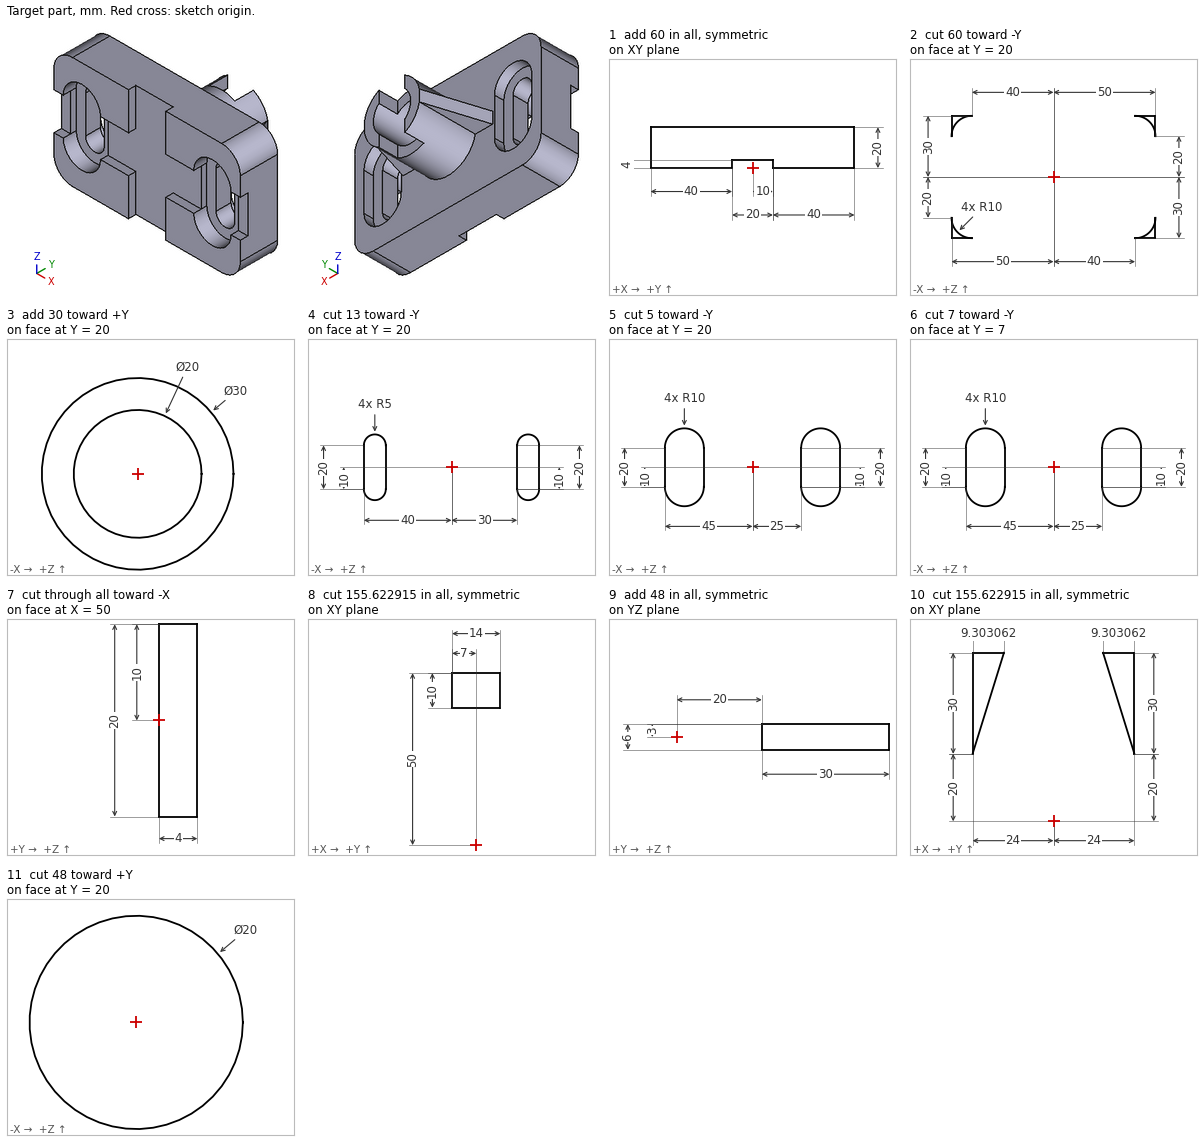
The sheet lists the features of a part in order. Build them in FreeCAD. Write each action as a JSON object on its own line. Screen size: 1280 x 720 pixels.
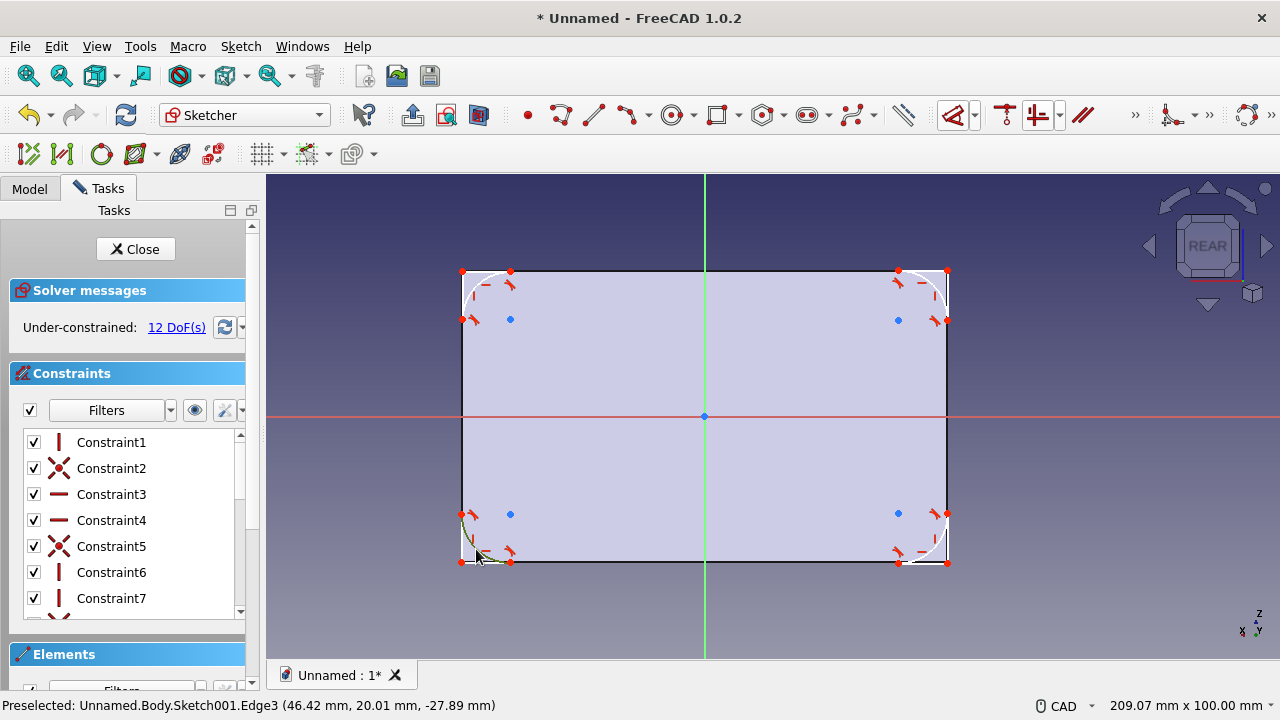
{"action": "left_click", "coordinate": [933, 549]}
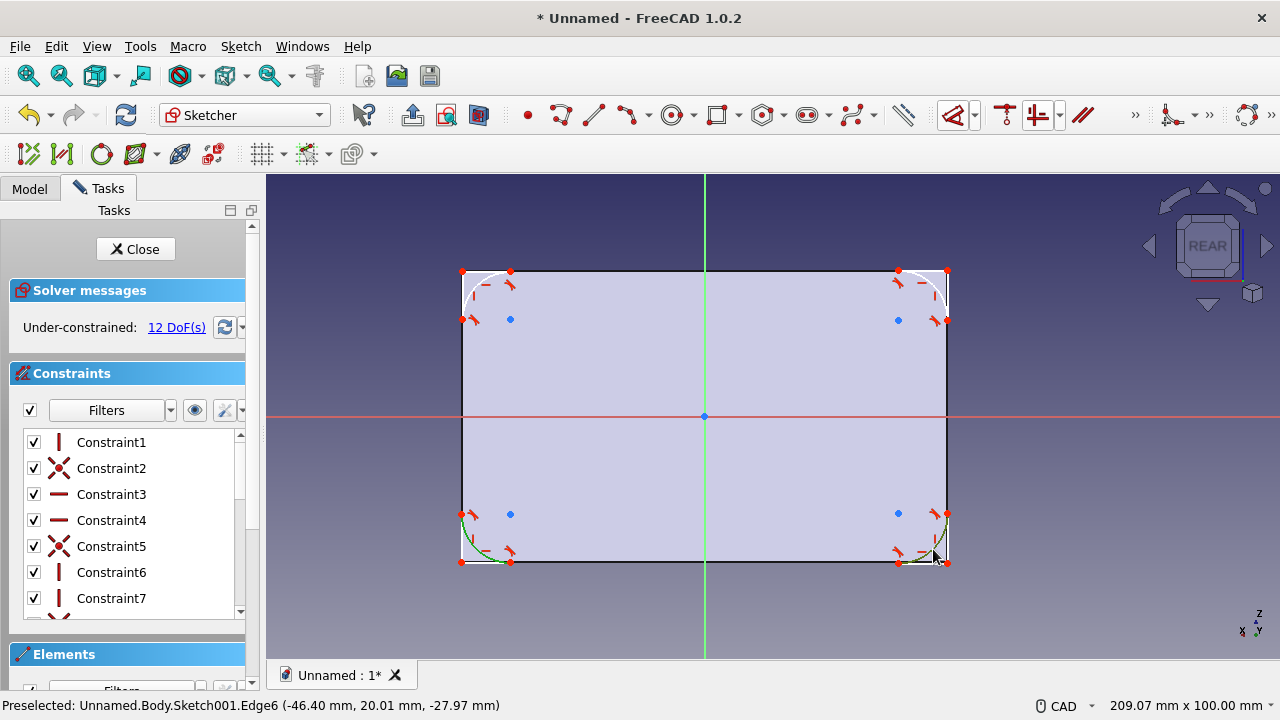
{"action": "left_click", "coordinate": [933, 285]}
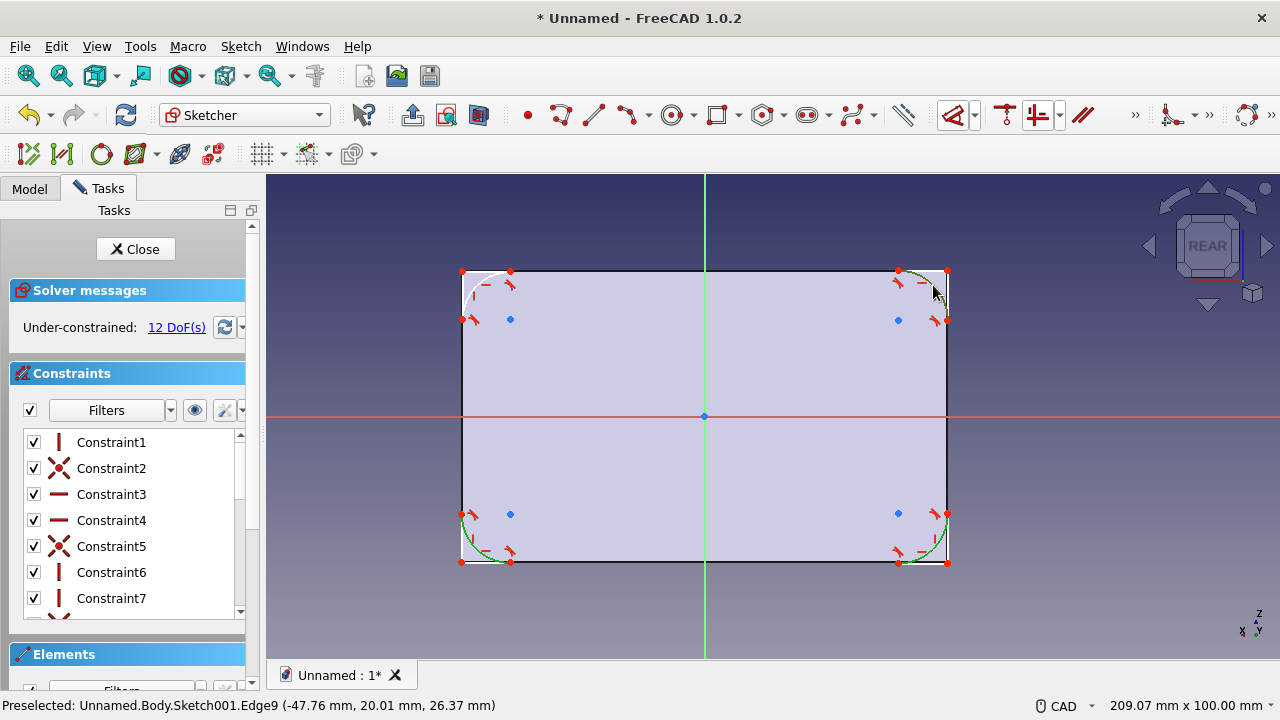
{"action": "left_click", "coordinate": [477, 286]}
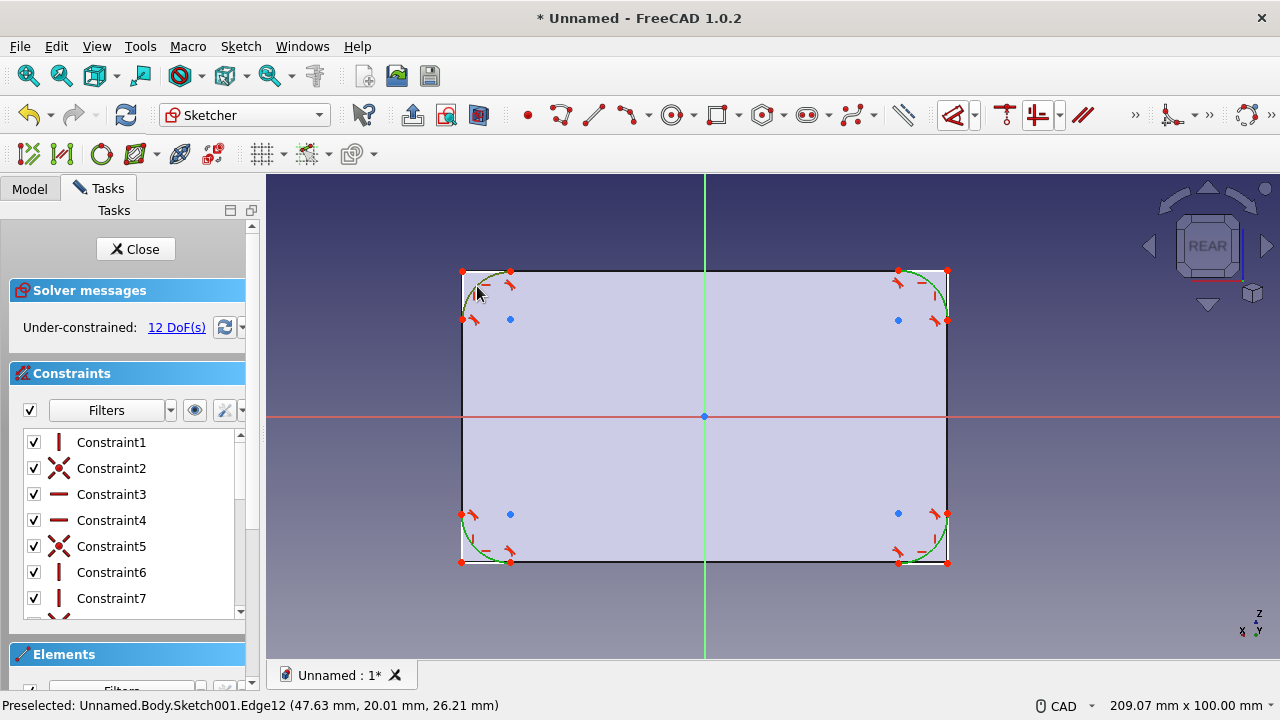
{"action": "key", "text": "e"}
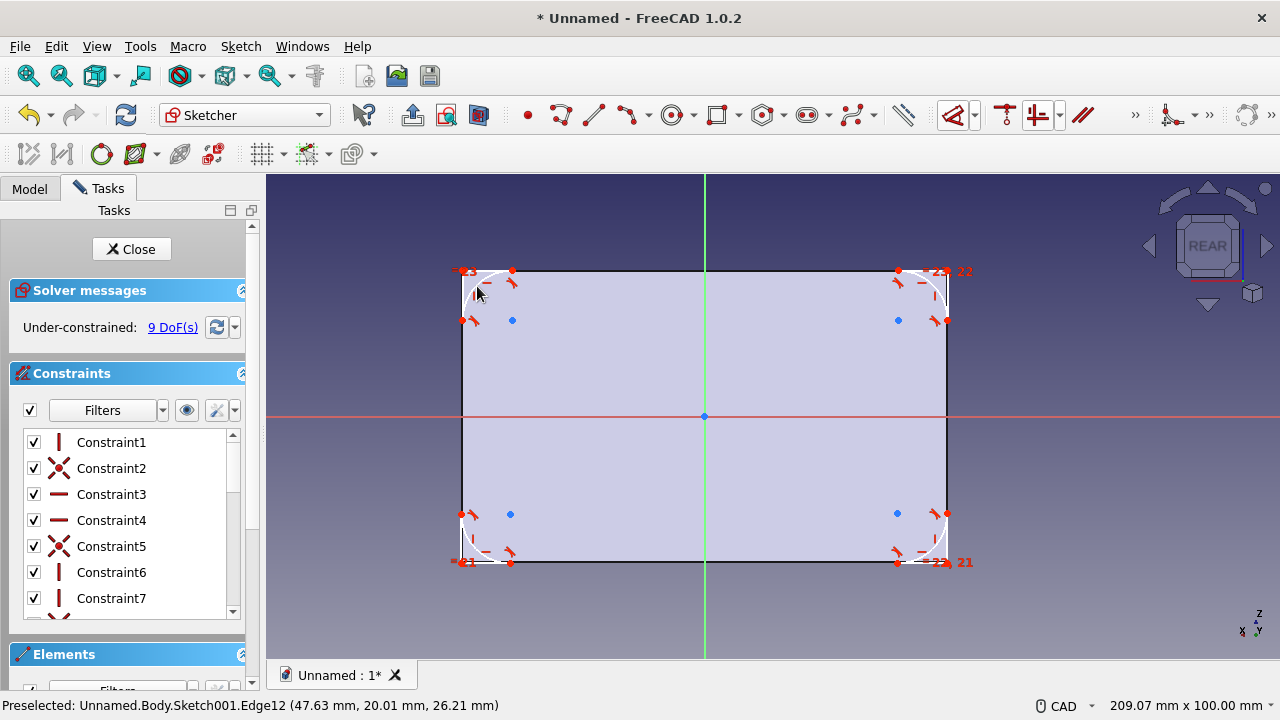
{"action": "left_click", "coordinate": [476, 549]}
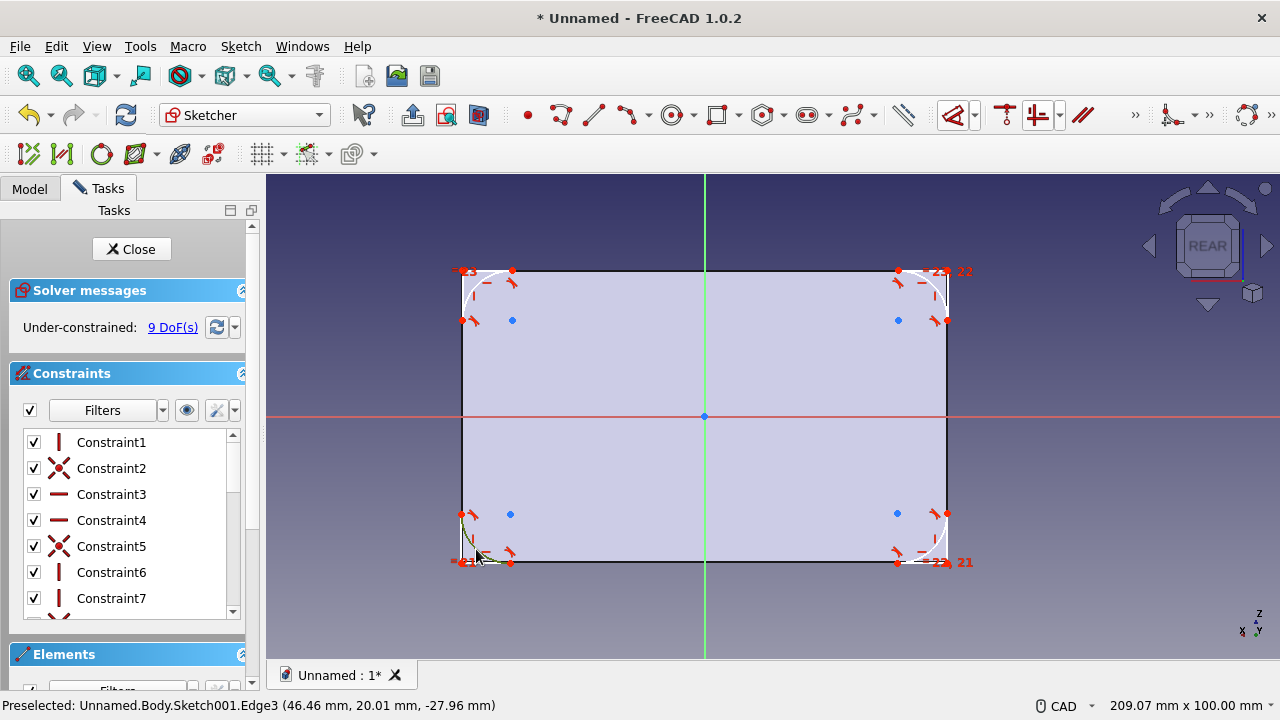
{"action": "key", "text": "k r"}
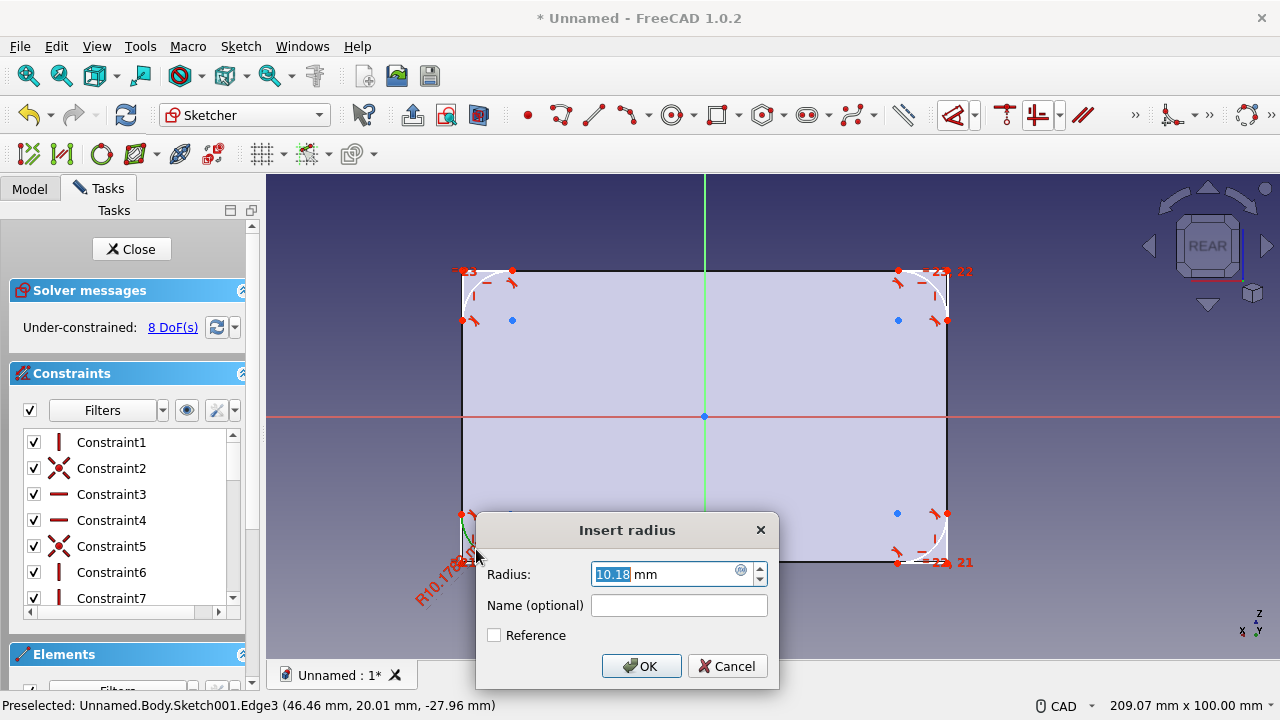
{"action": "type", "text": "10"}
{"action": "key", "text": "Return"}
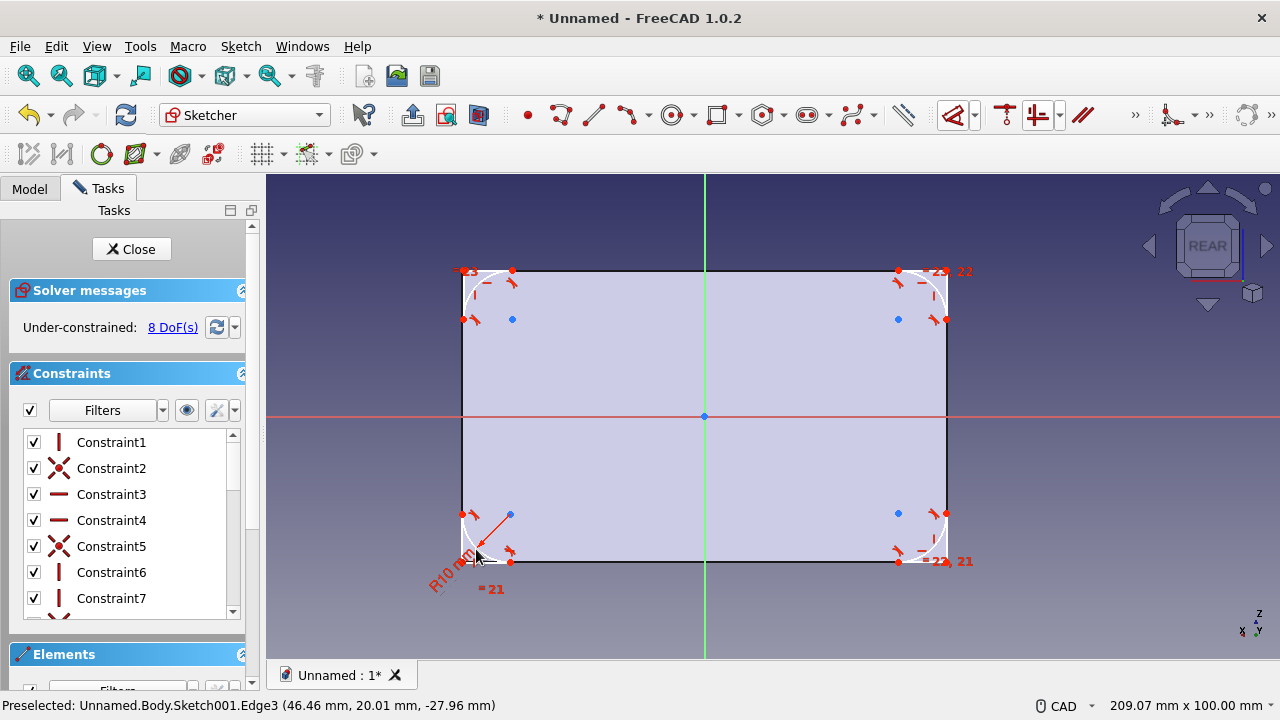
{"action": "left_click", "coordinate": [462, 514]}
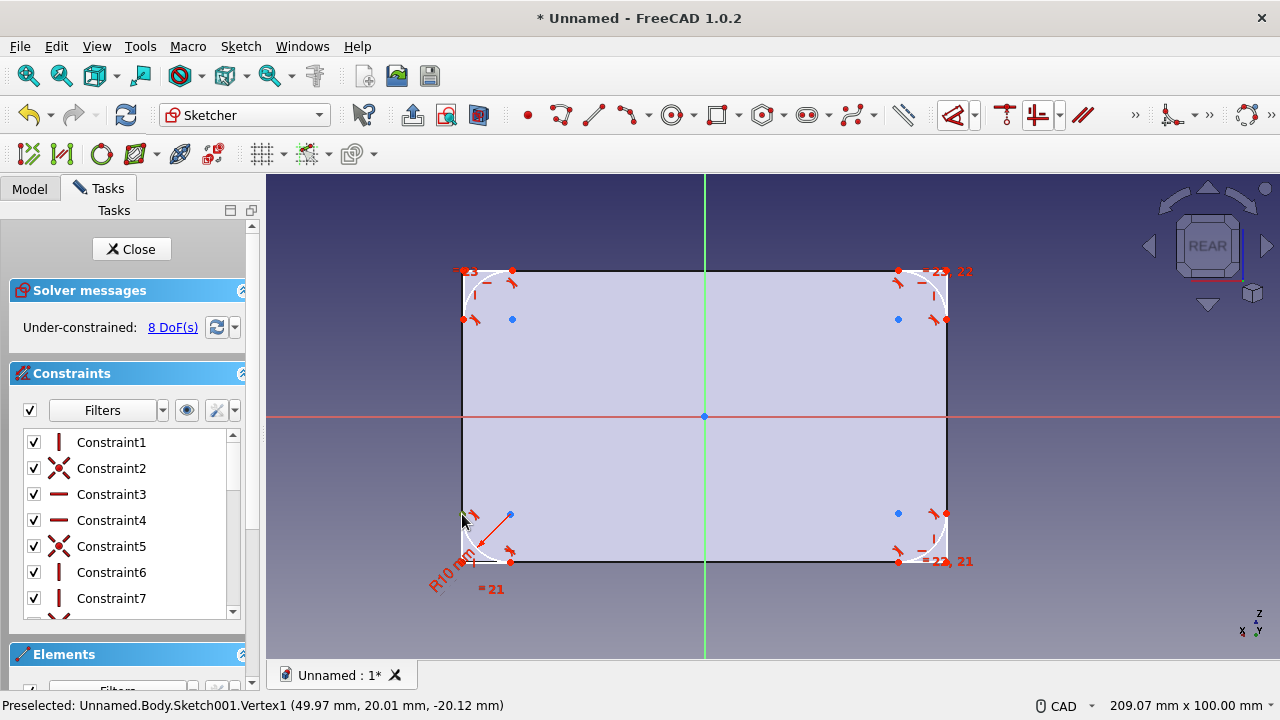
{"action": "key", "text": "l"}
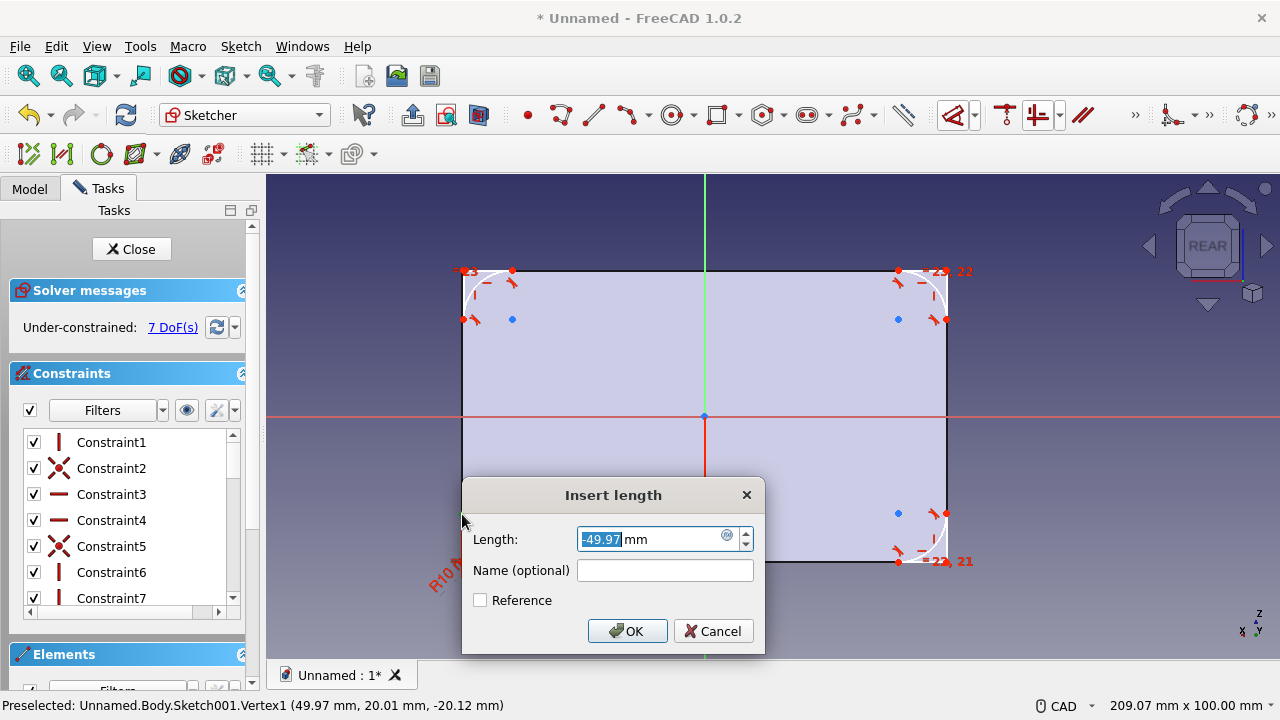
{"action": "type", "text": "-50"}
{"action": "key", "text": "Return"}